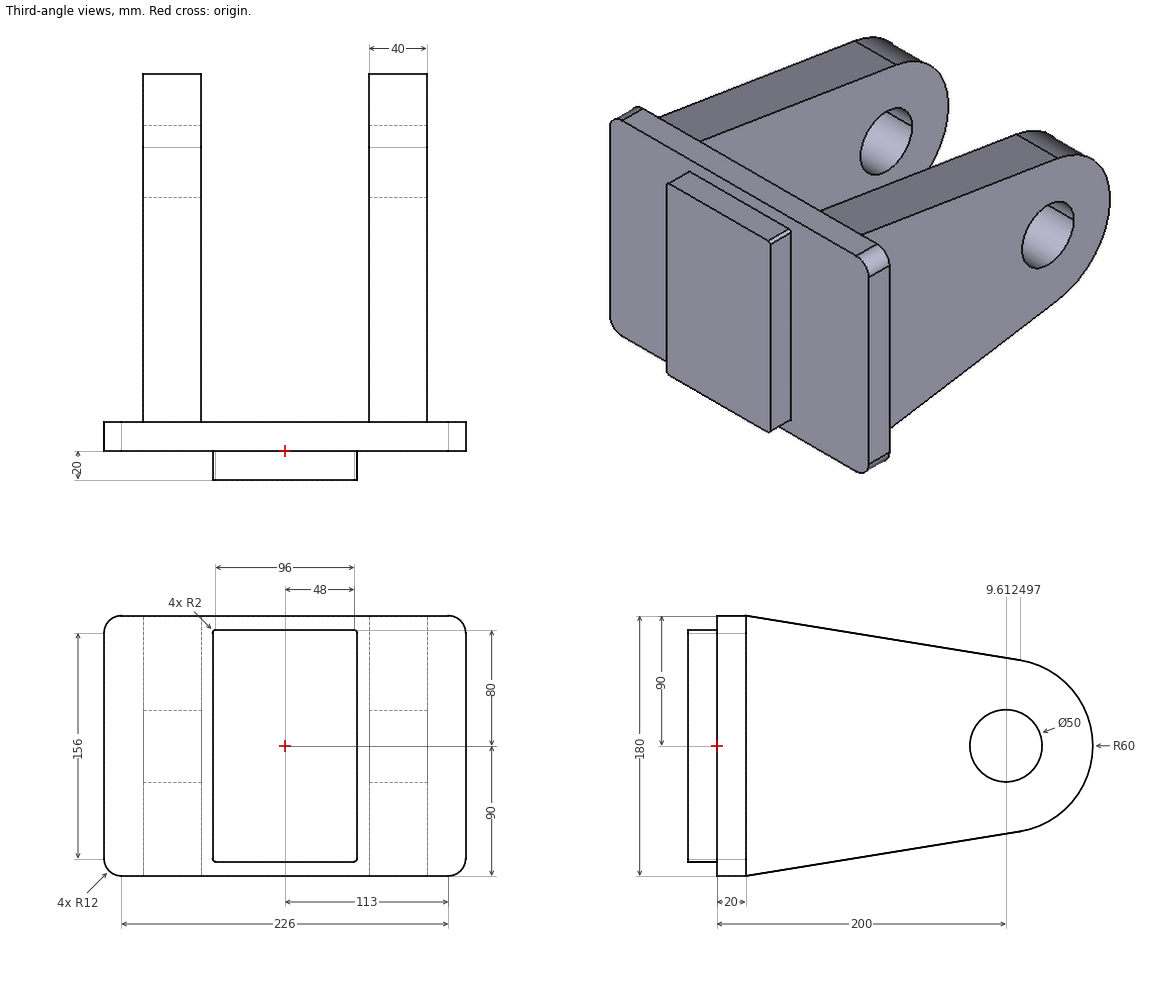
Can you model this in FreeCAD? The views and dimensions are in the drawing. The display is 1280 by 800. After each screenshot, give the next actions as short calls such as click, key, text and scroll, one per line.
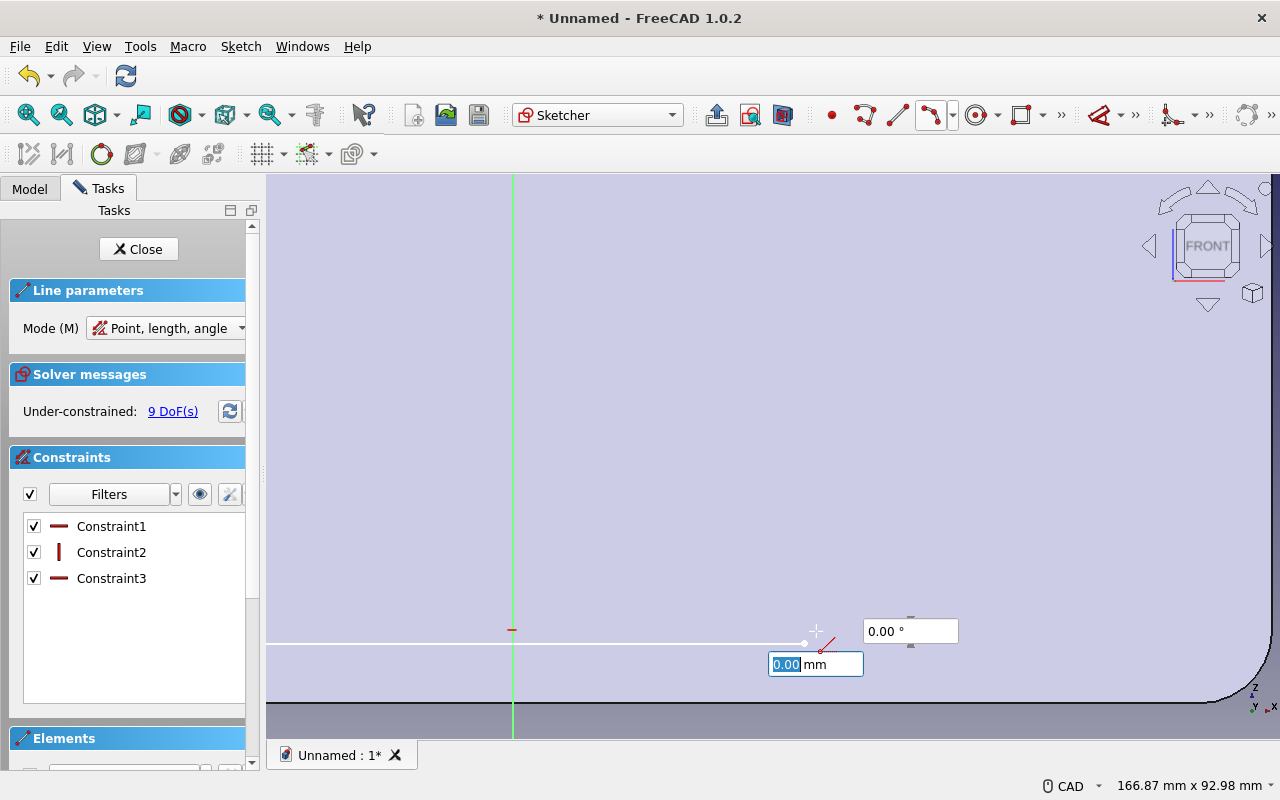
scroll(816, 631, down, 5)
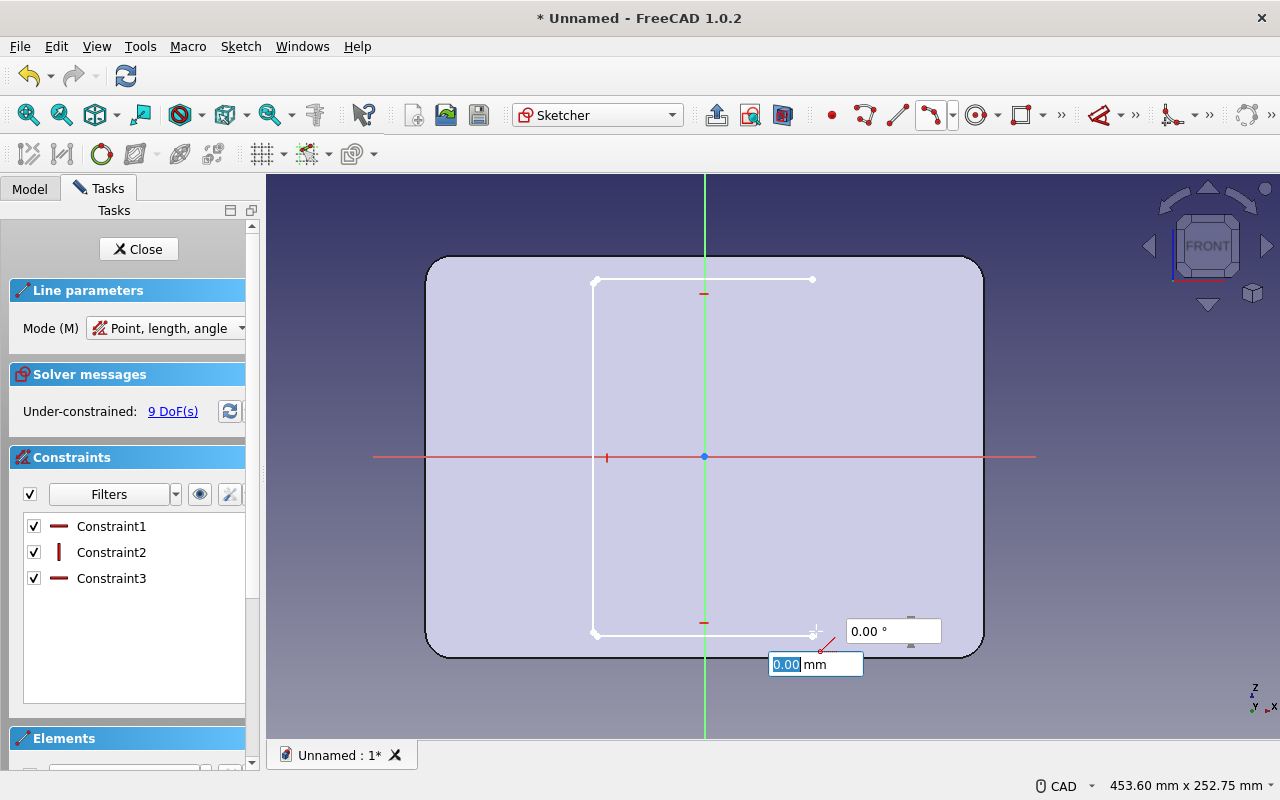
scroll(816, 283, up, 5)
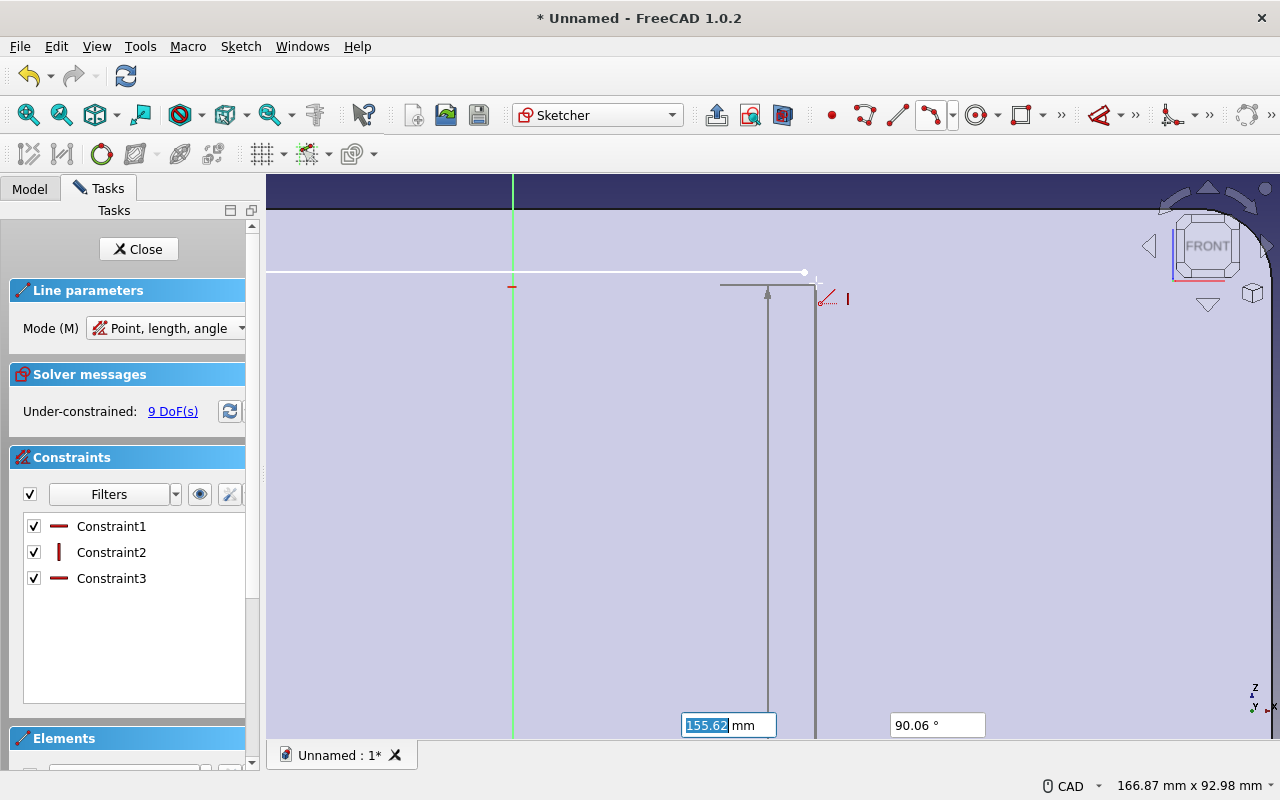
click(816, 282)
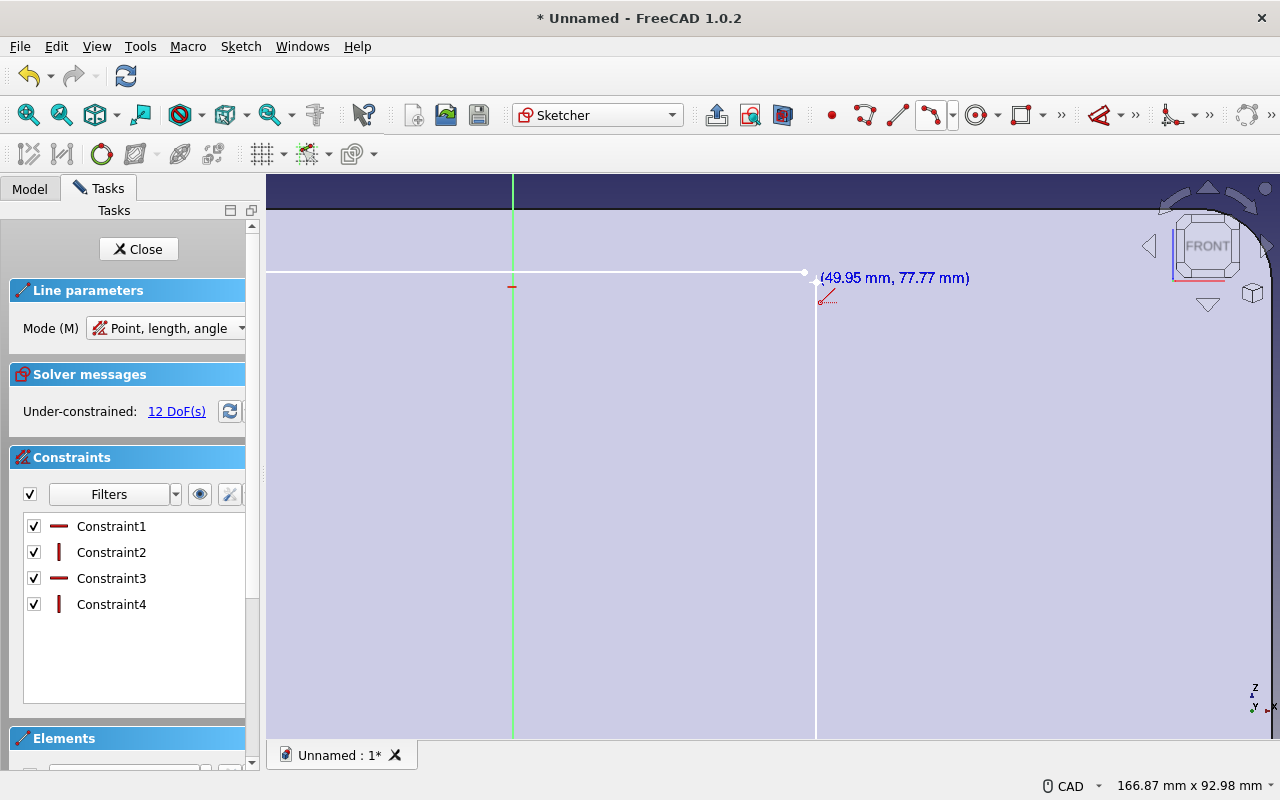
click(930, 116)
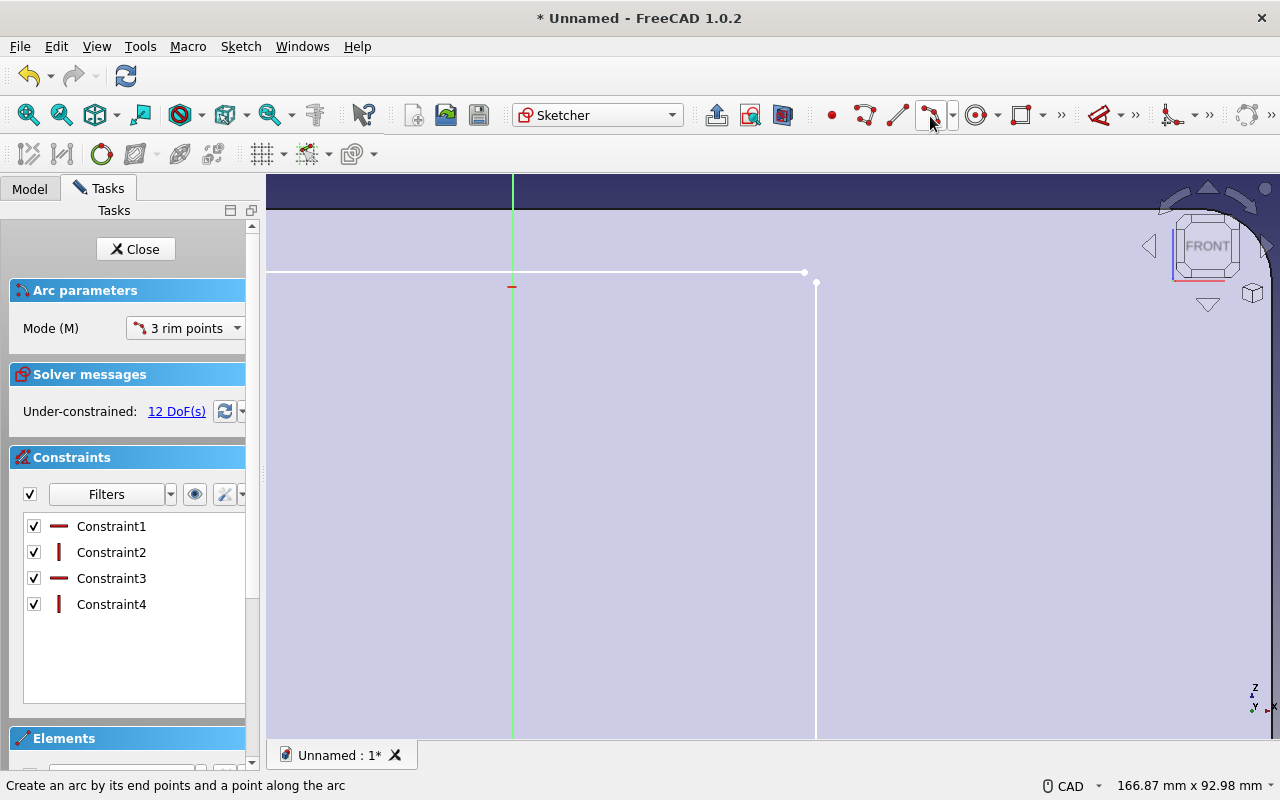
scroll(816, 282, down, 5)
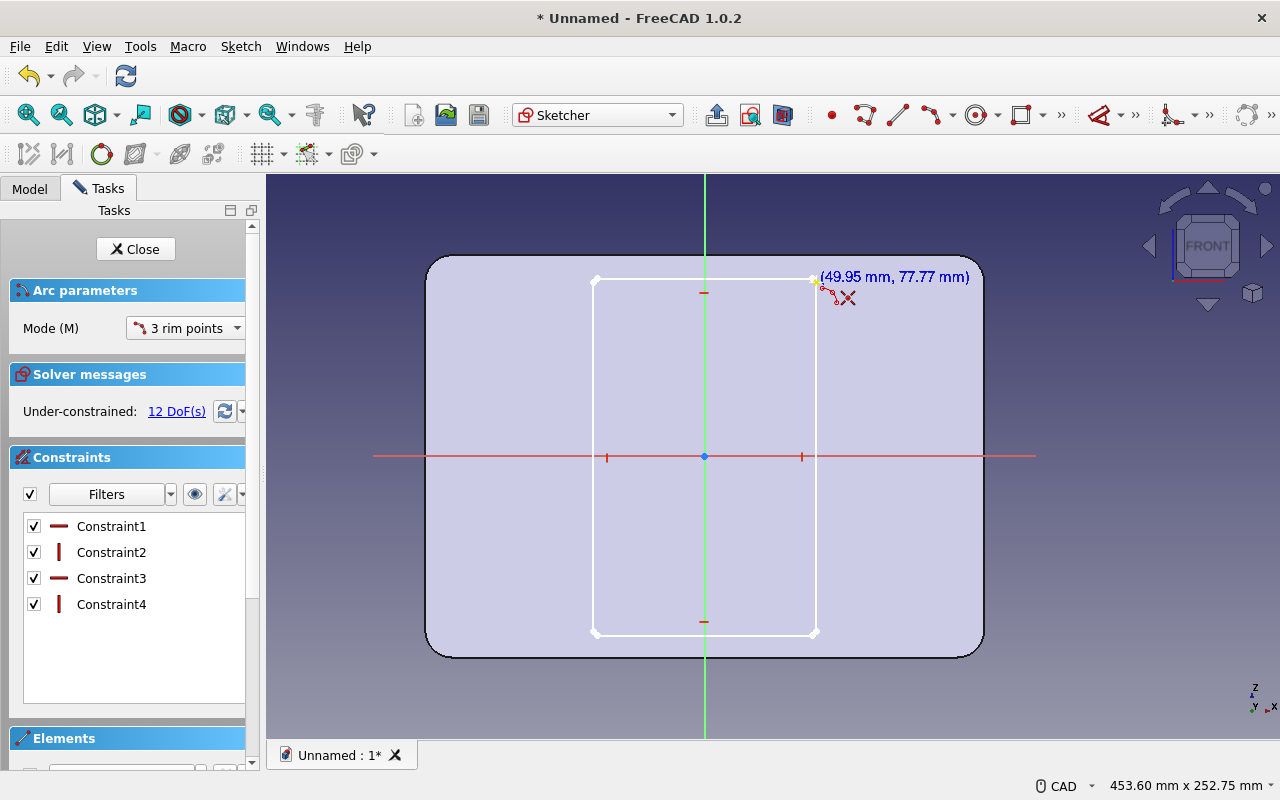
scroll(597, 277, up, 5)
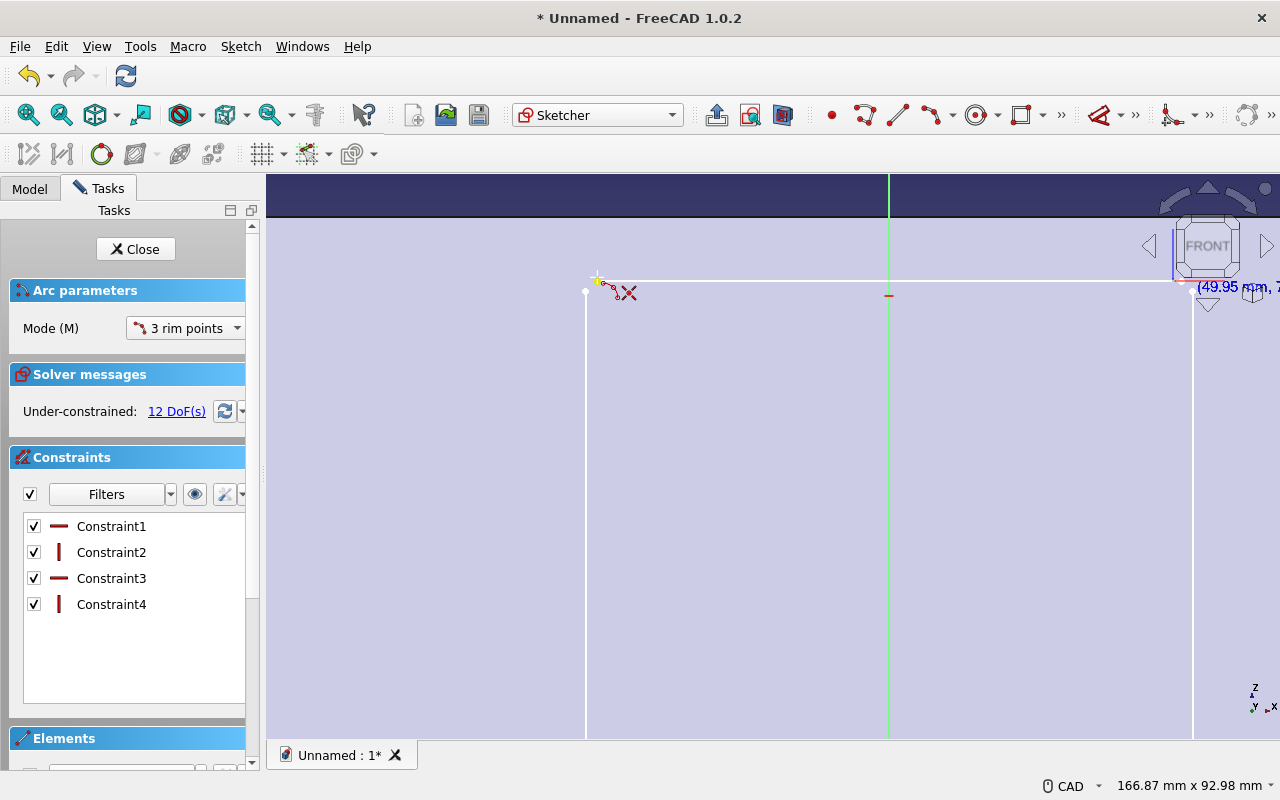
click(597, 281)
click(586, 292)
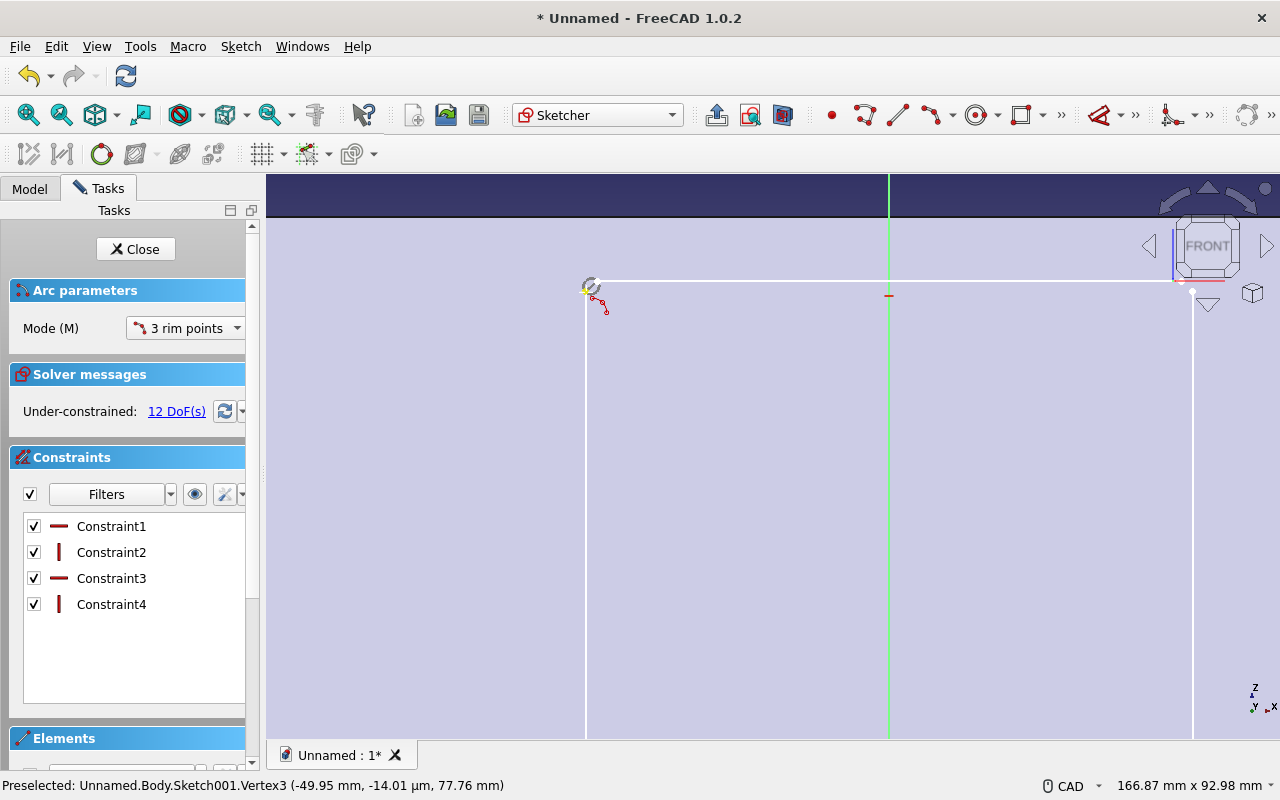
scroll(589, 282, up, 8)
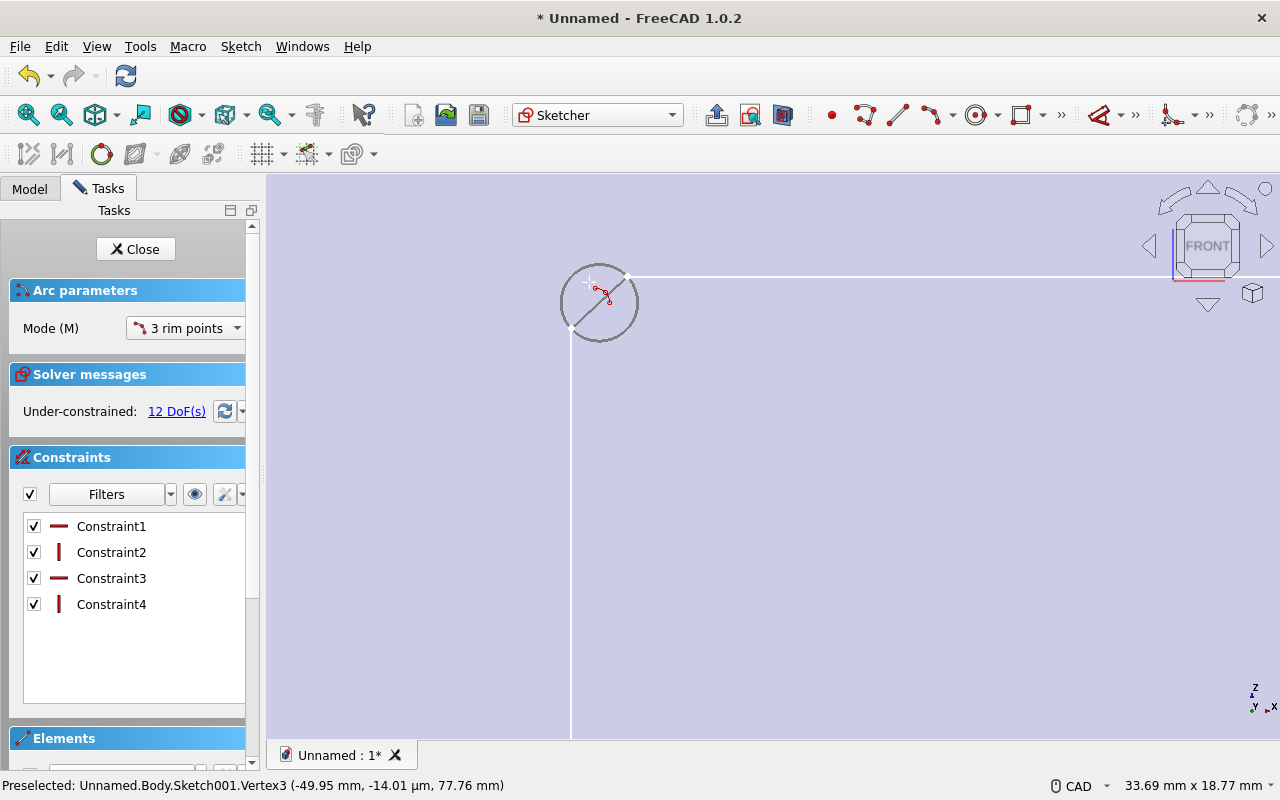
click(587, 279)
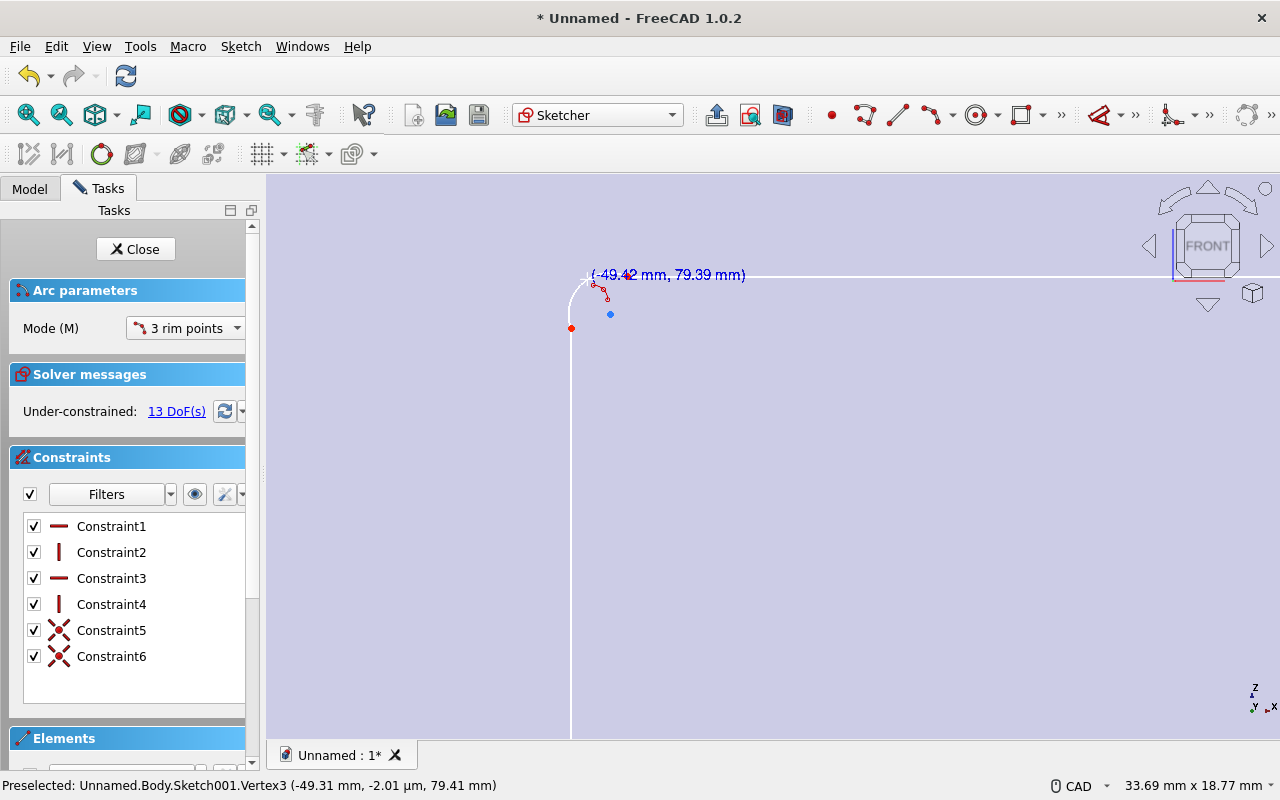
scroll(595, 279, down, 13)